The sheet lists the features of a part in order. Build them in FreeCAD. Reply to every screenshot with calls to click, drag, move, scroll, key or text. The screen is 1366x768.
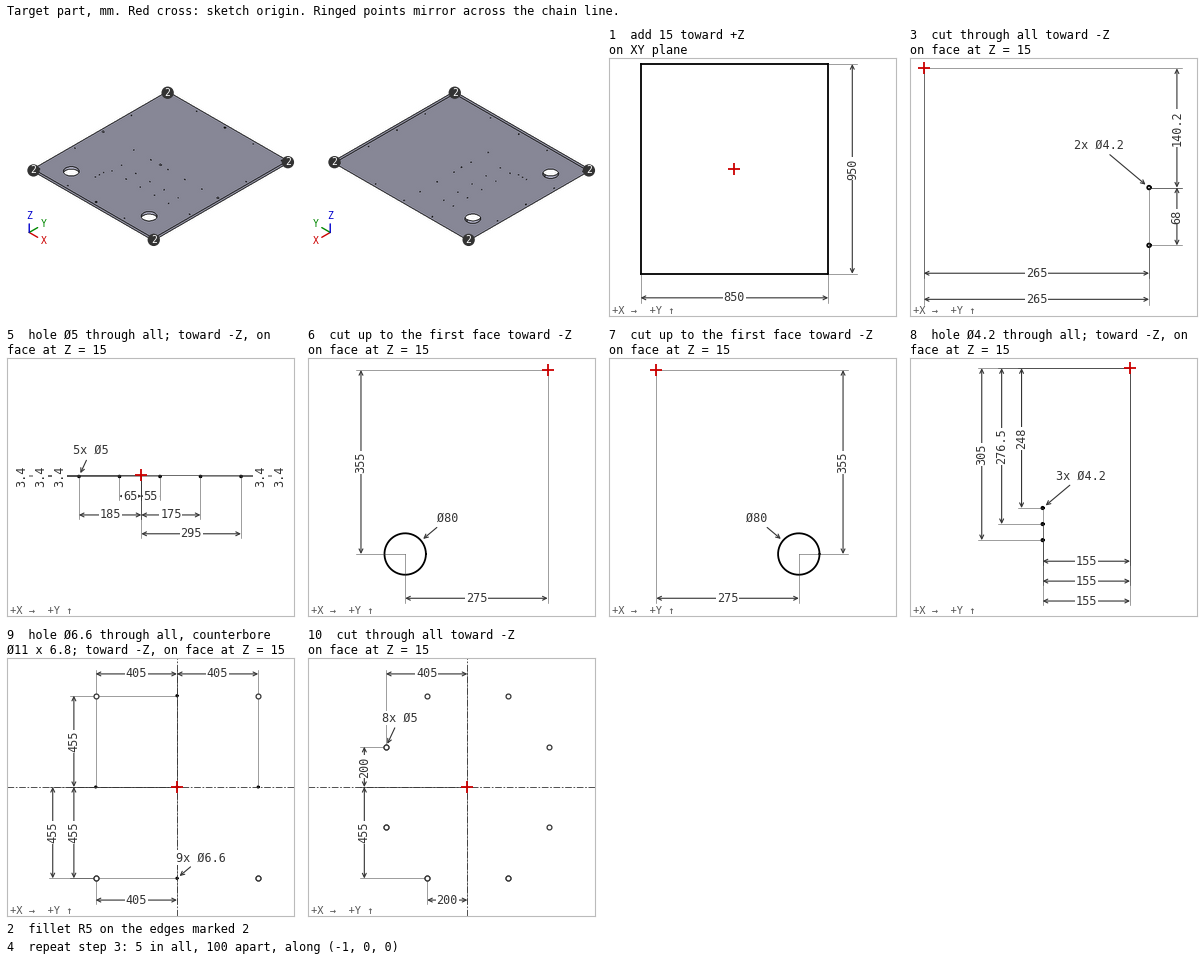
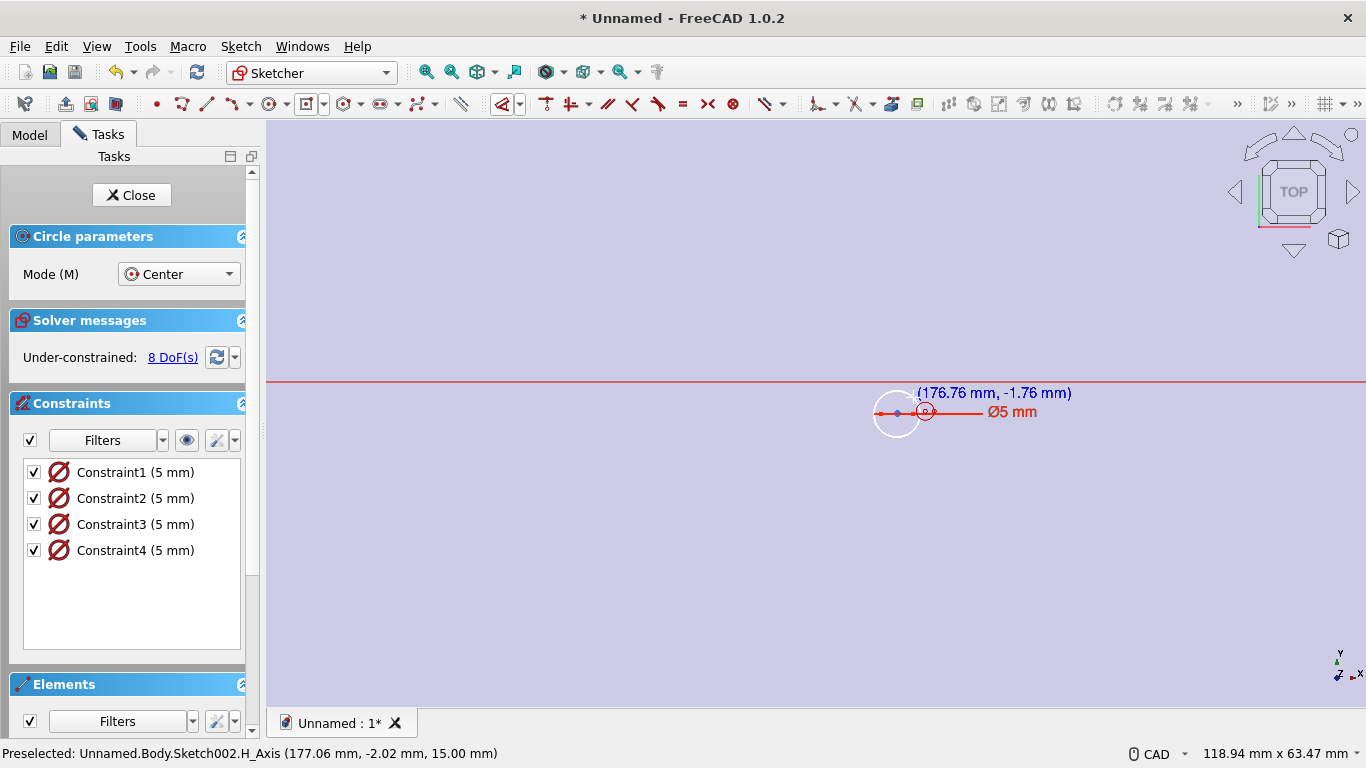
scroll(898, 414, down, 10)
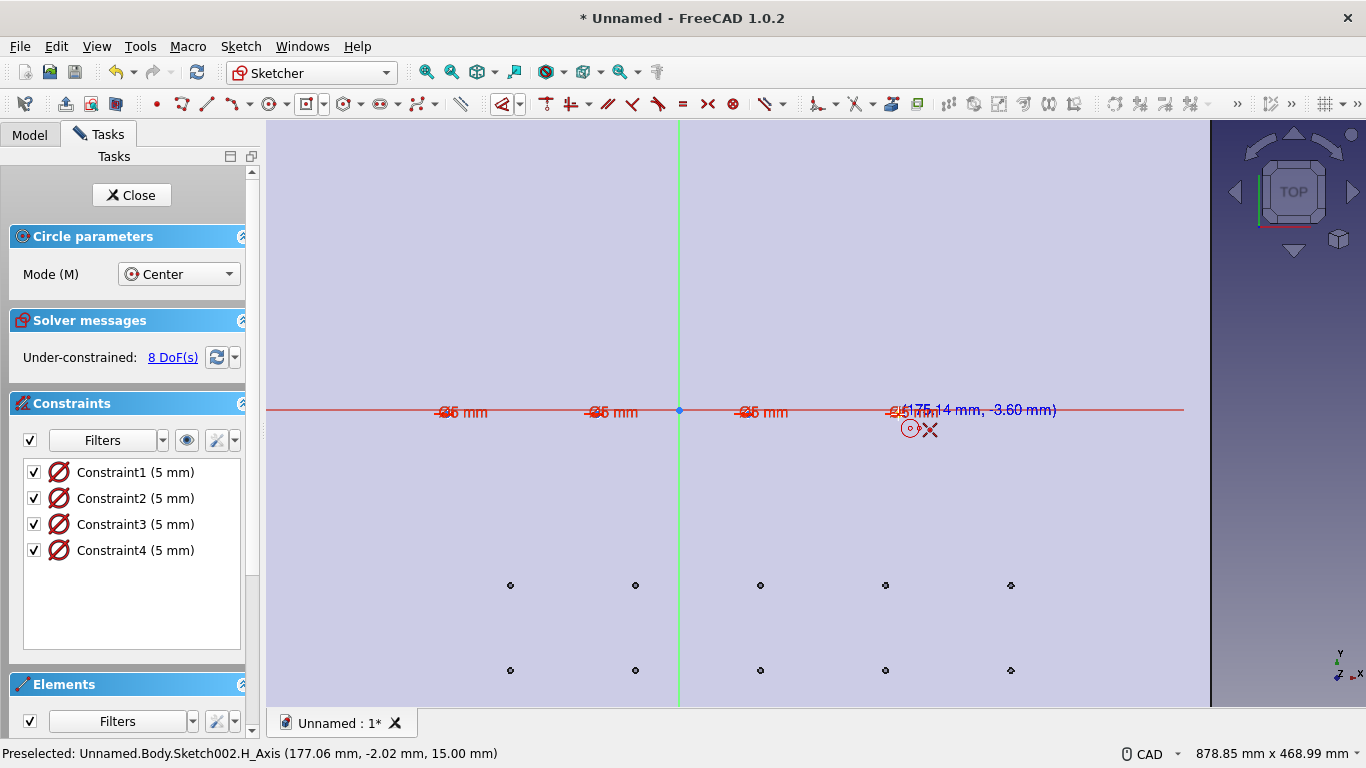
scroll(1049, 414, up, 10)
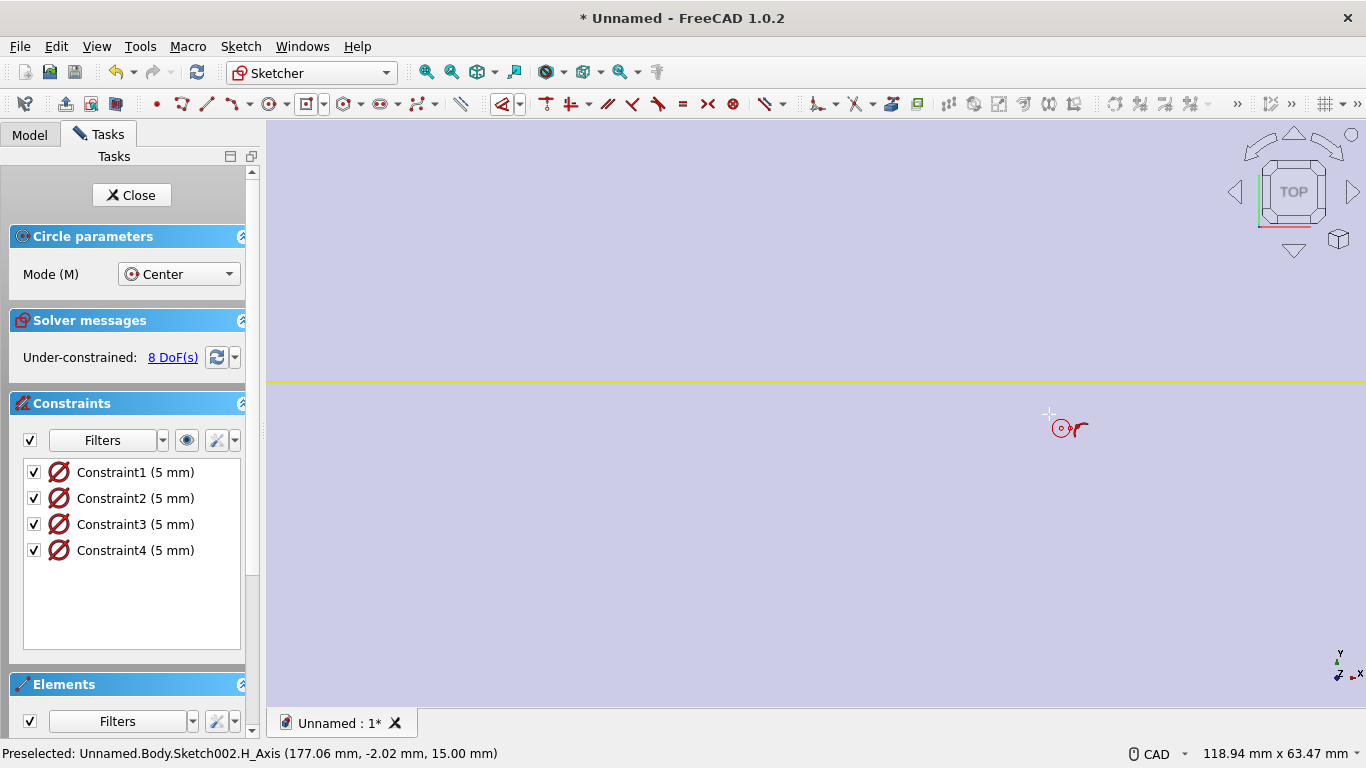
click(1041, 413)
move(1057, 397)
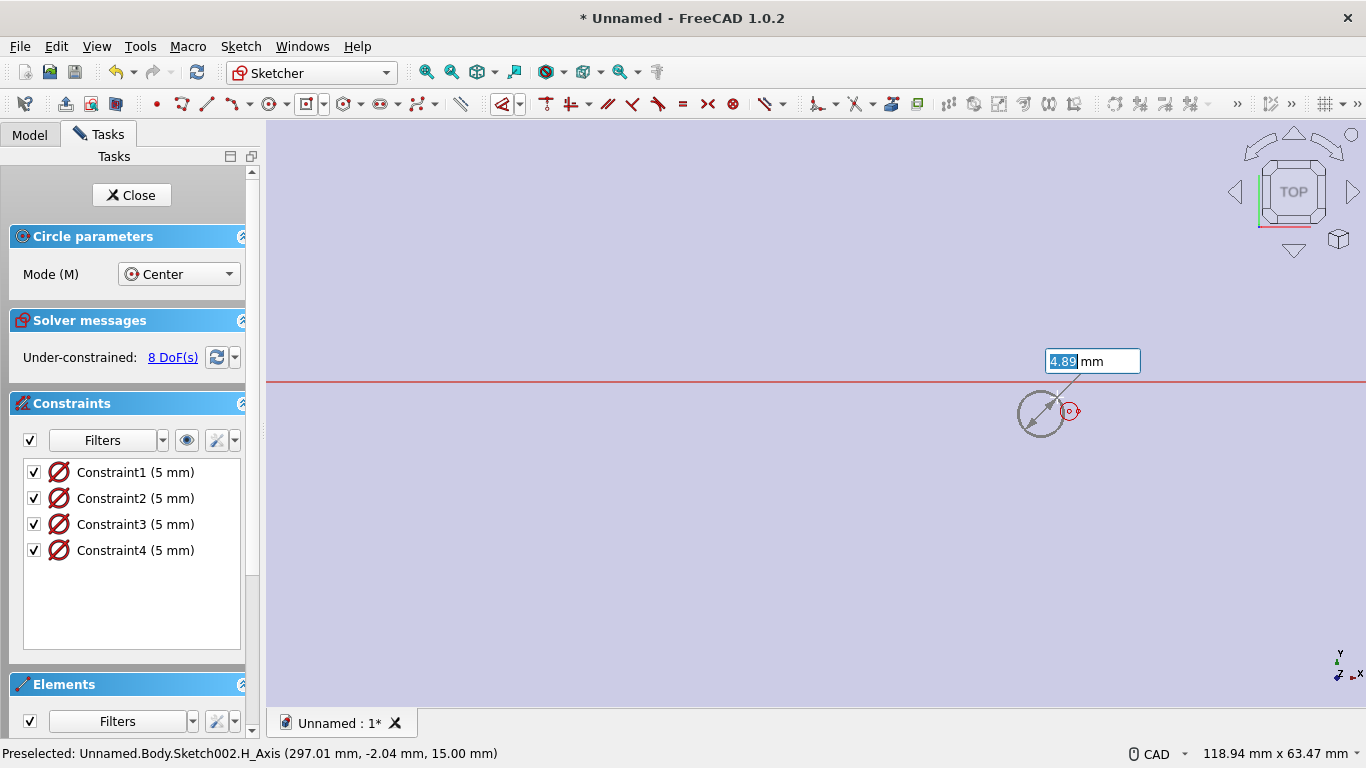
text(5)
key(Return)
key(Escape)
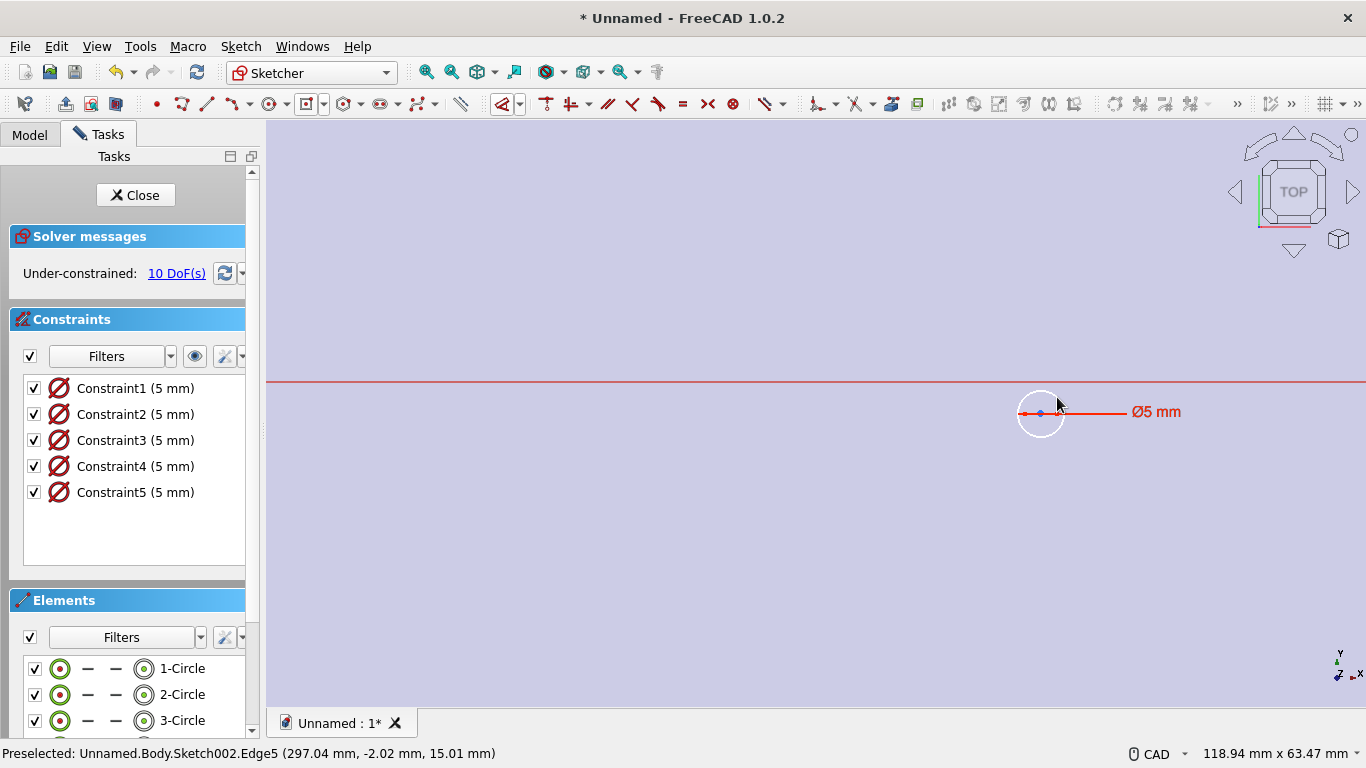
scroll(1049, 414, down, 10)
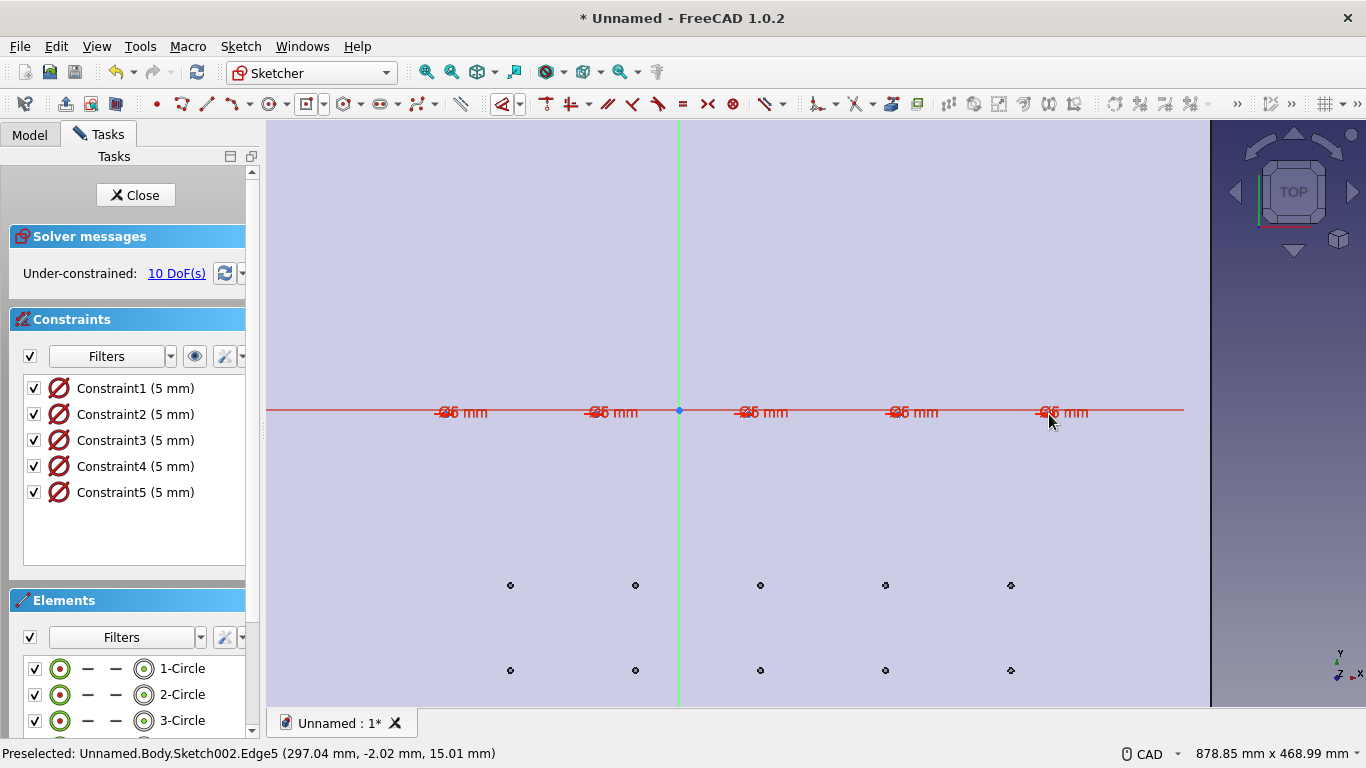
click(598, 414)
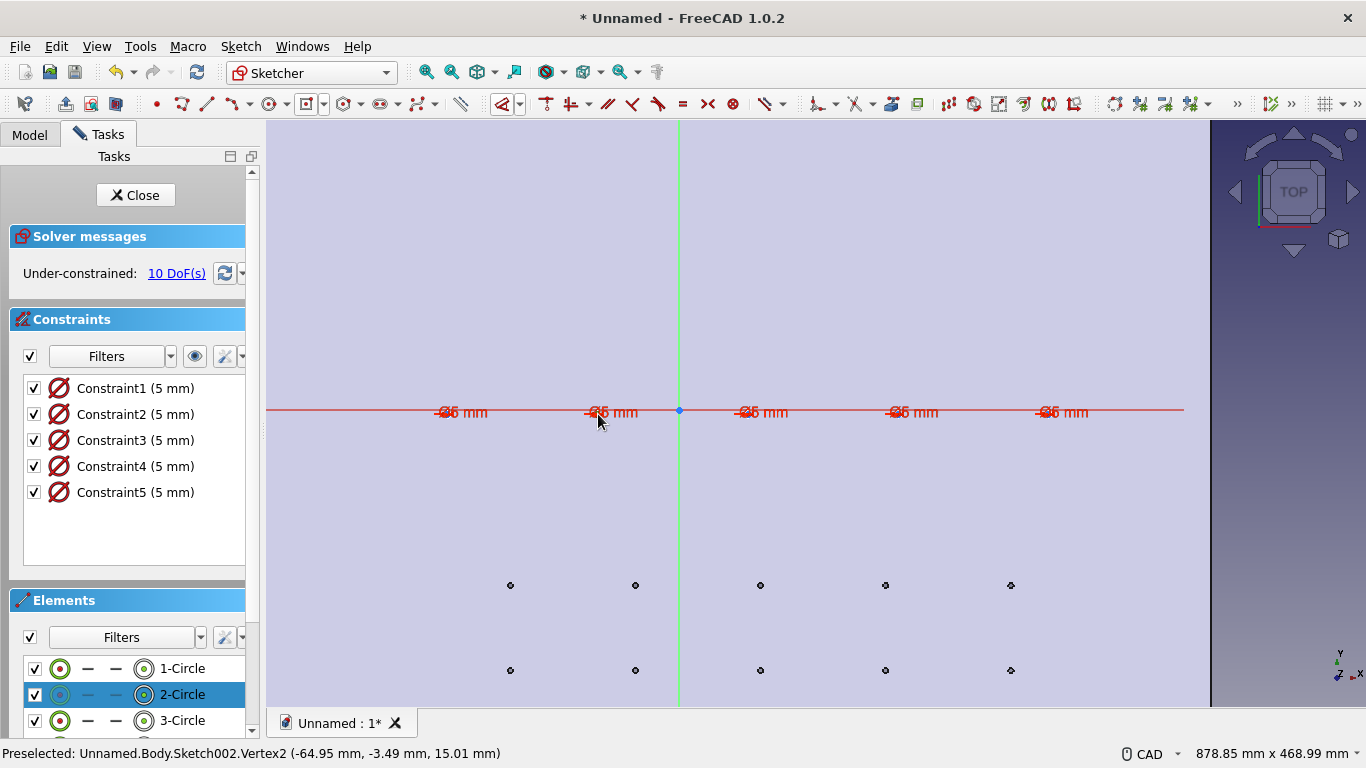
click(520, 104)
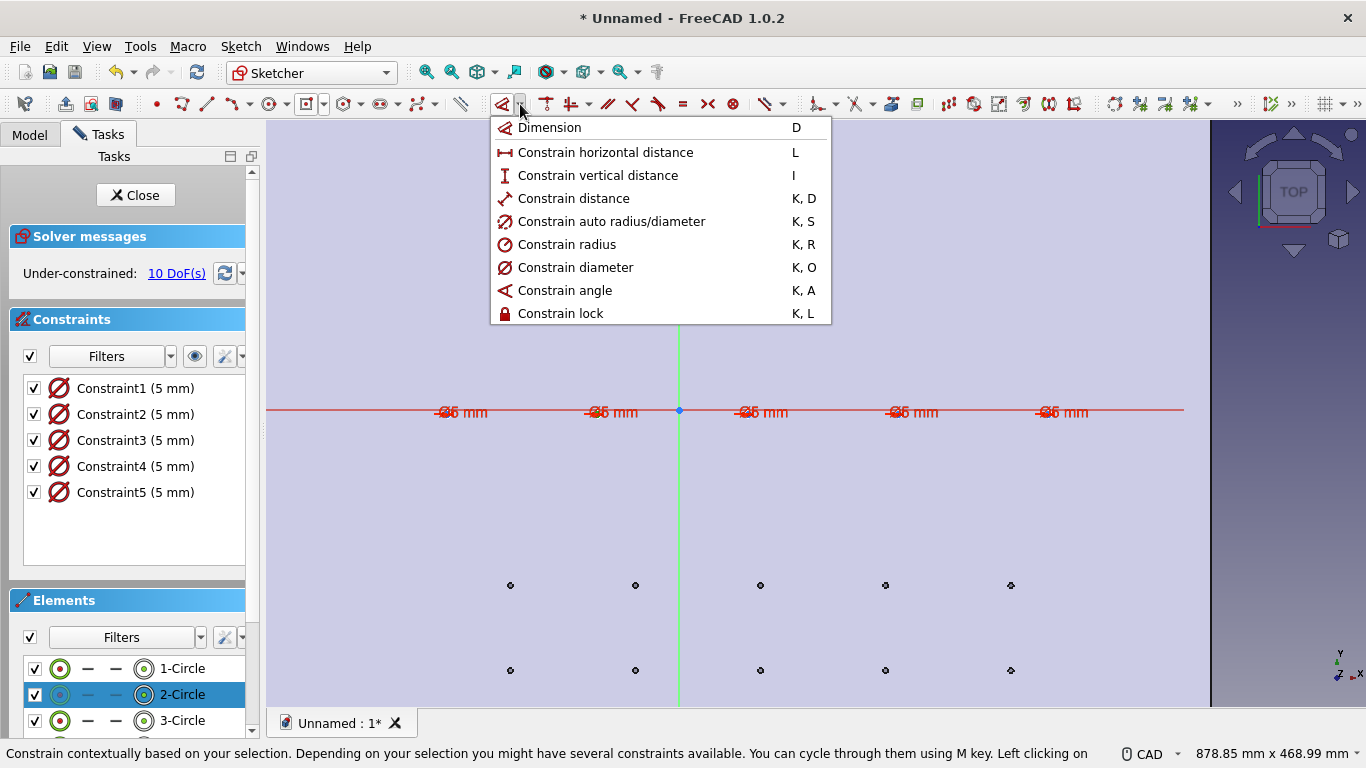
click(661, 152)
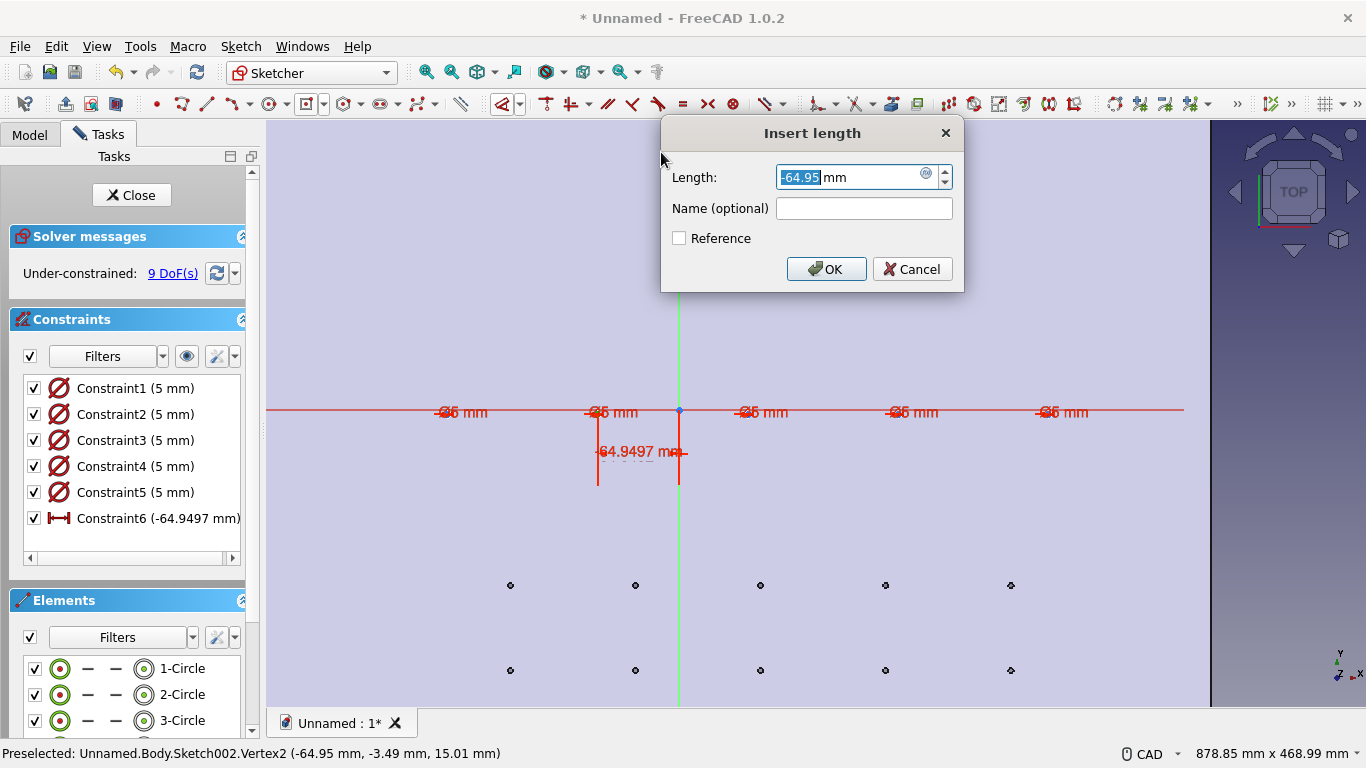
text(-65)
key(Return)